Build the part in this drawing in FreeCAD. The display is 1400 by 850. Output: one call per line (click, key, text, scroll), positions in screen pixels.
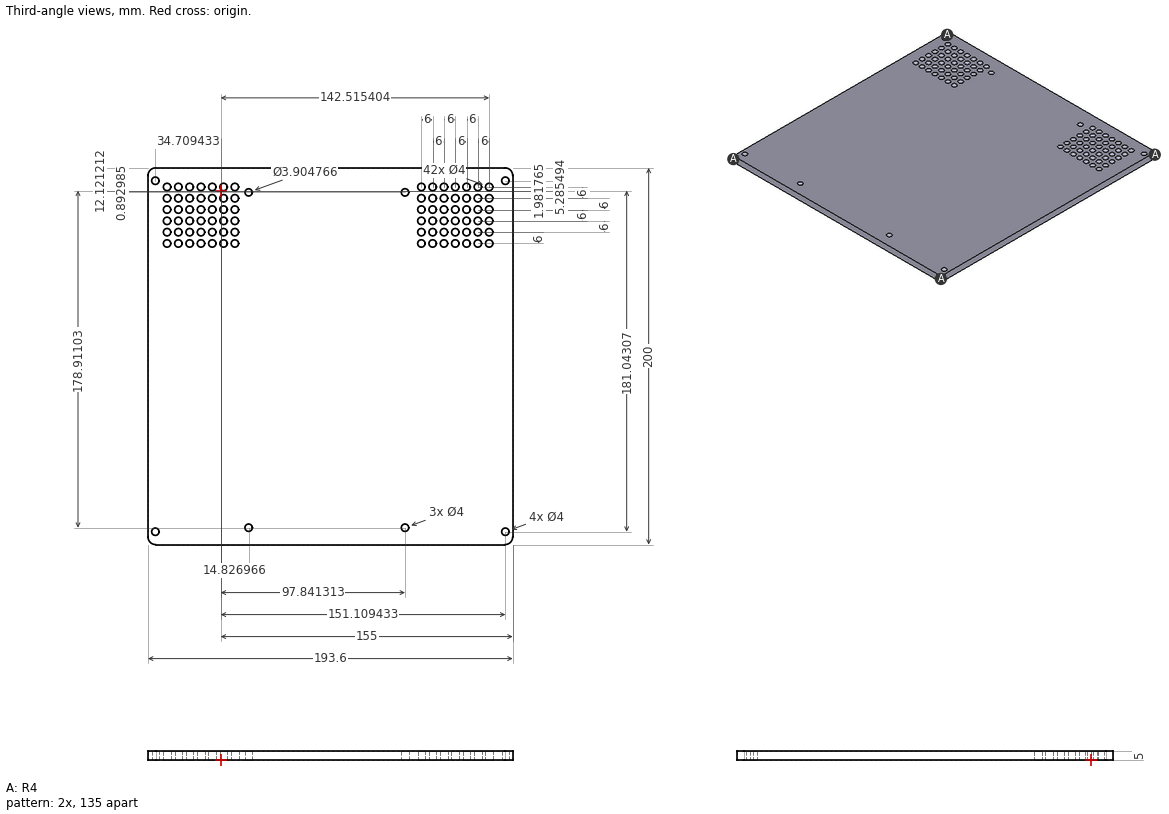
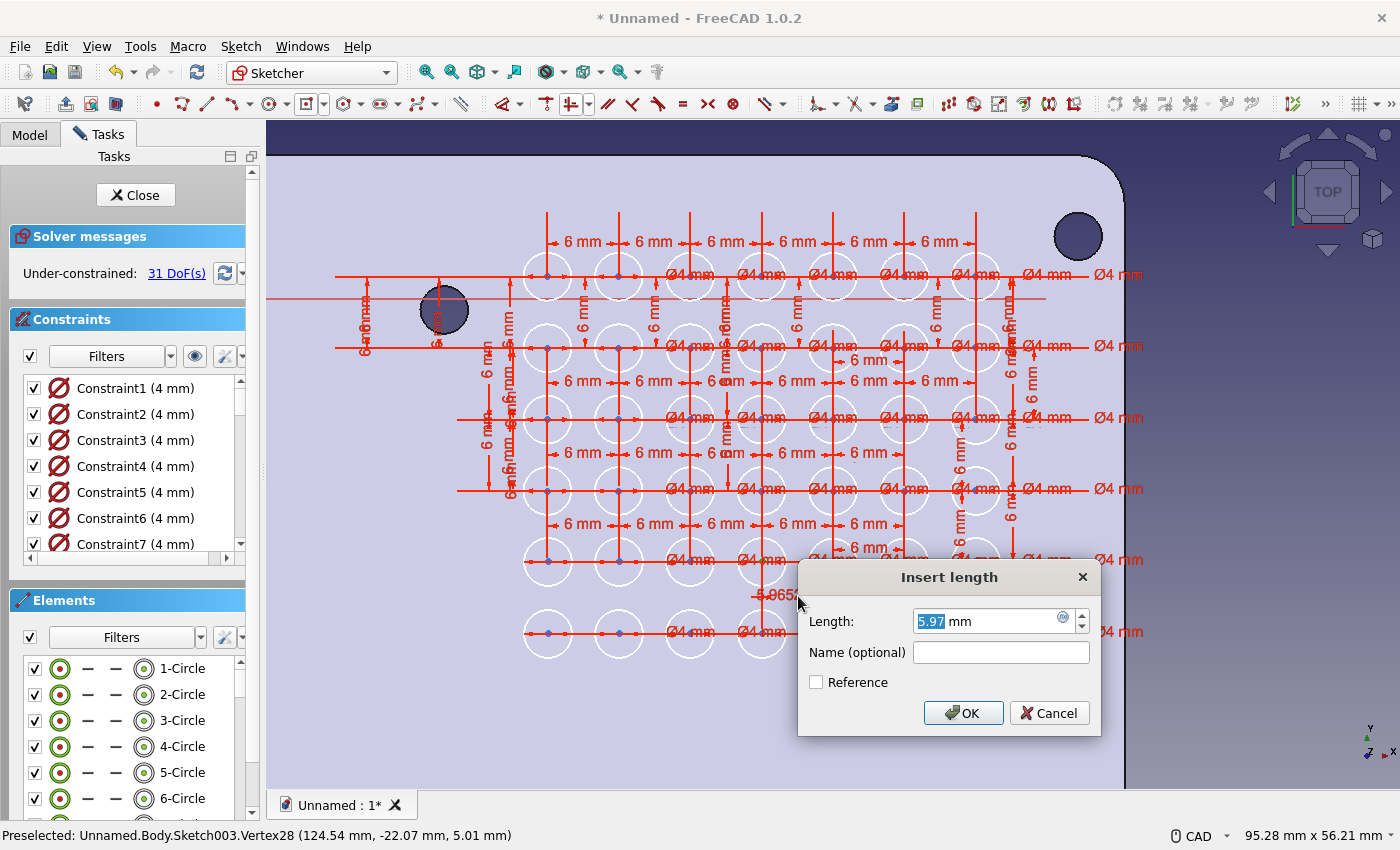
text(6)
key(Return)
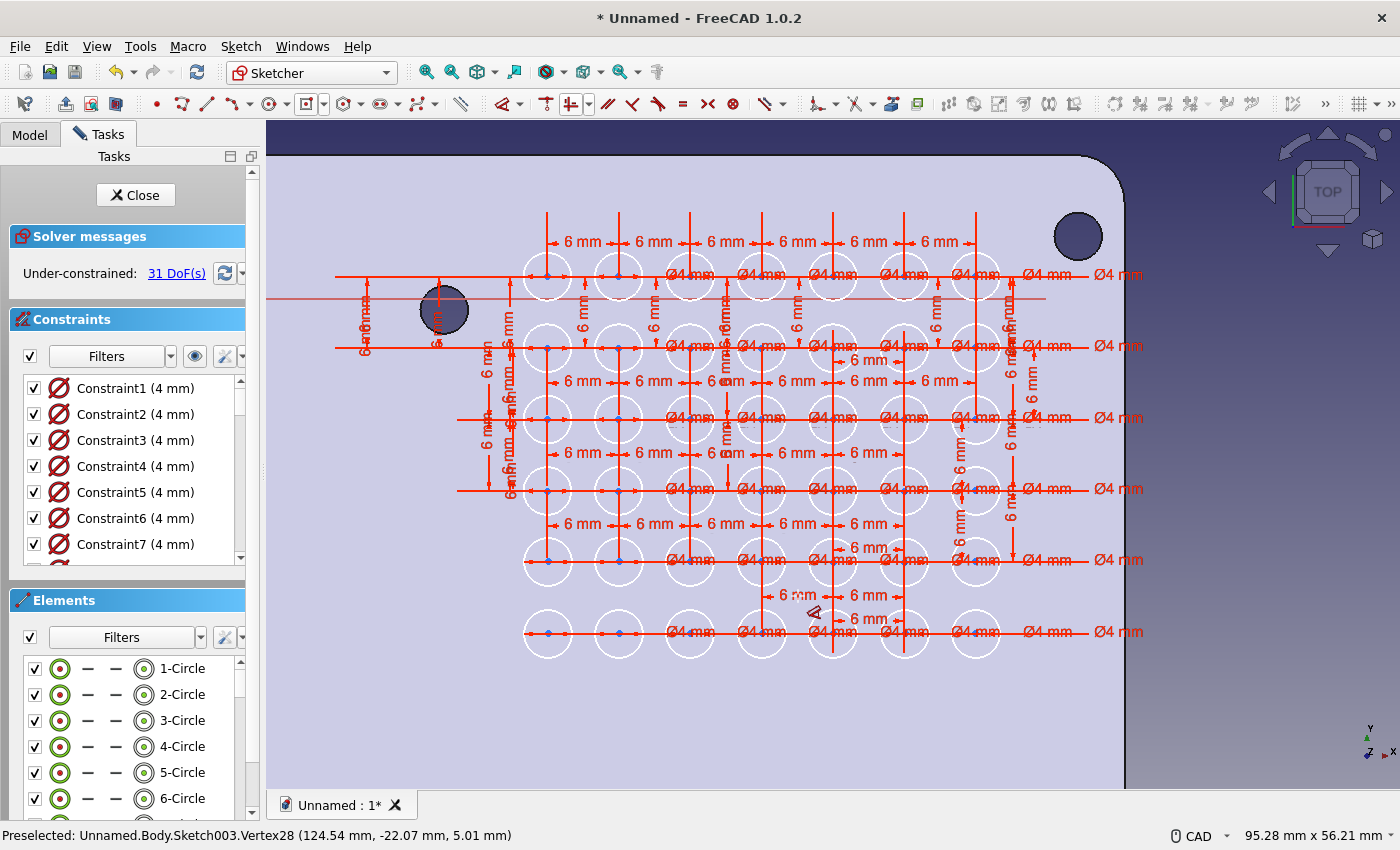
click(762, 491)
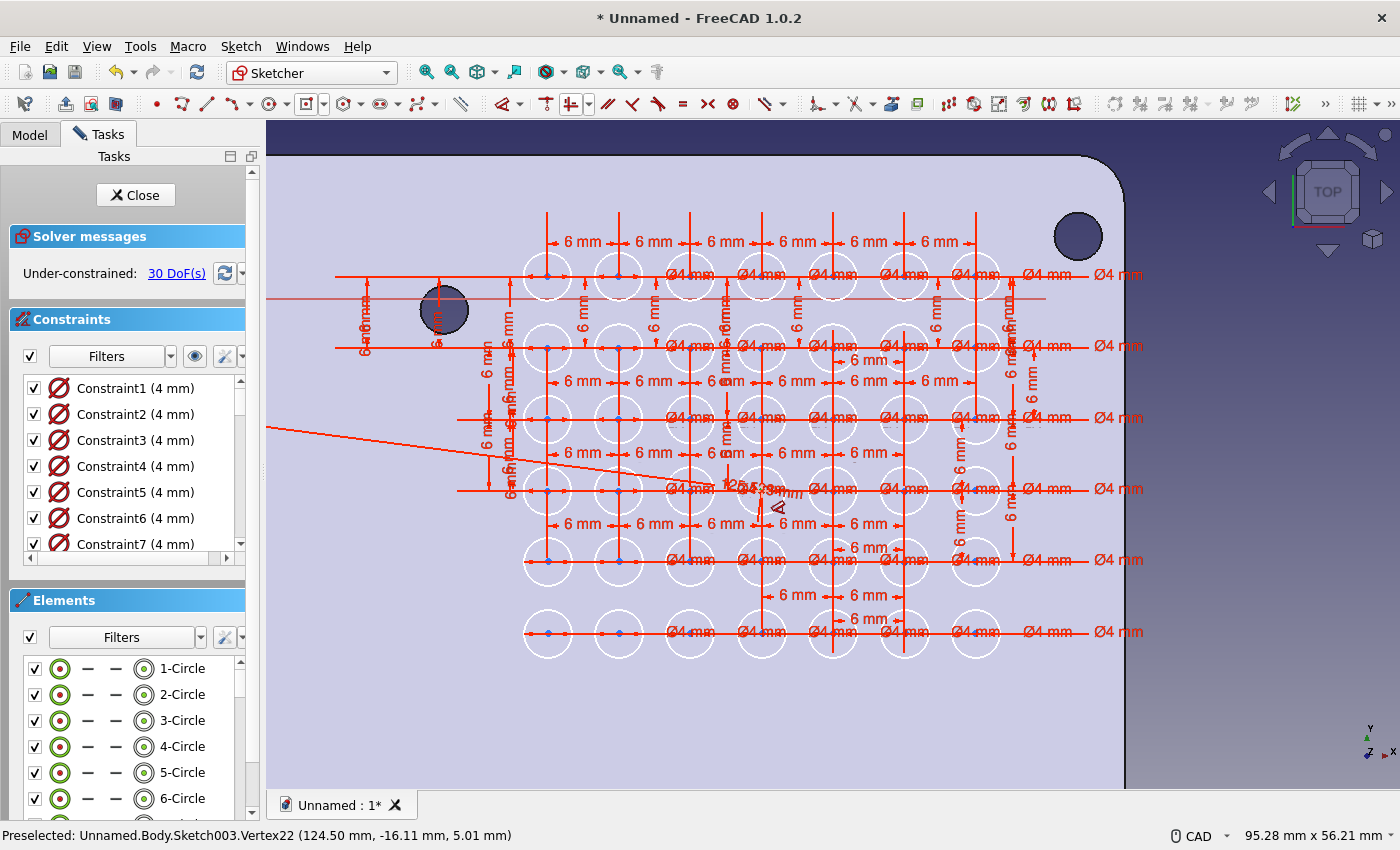
click(762, 562)
click(728, 510)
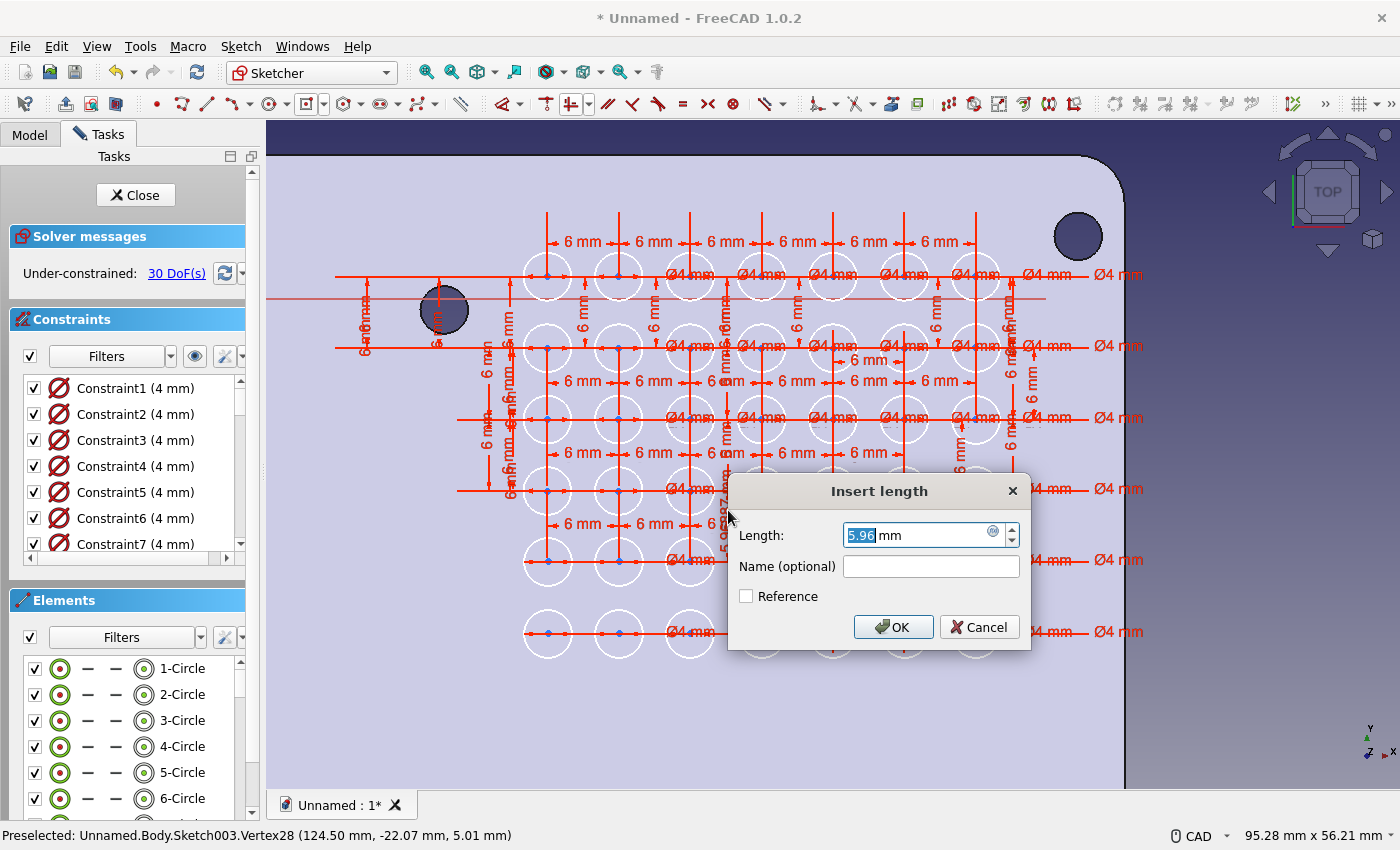
text(6)
key(Return)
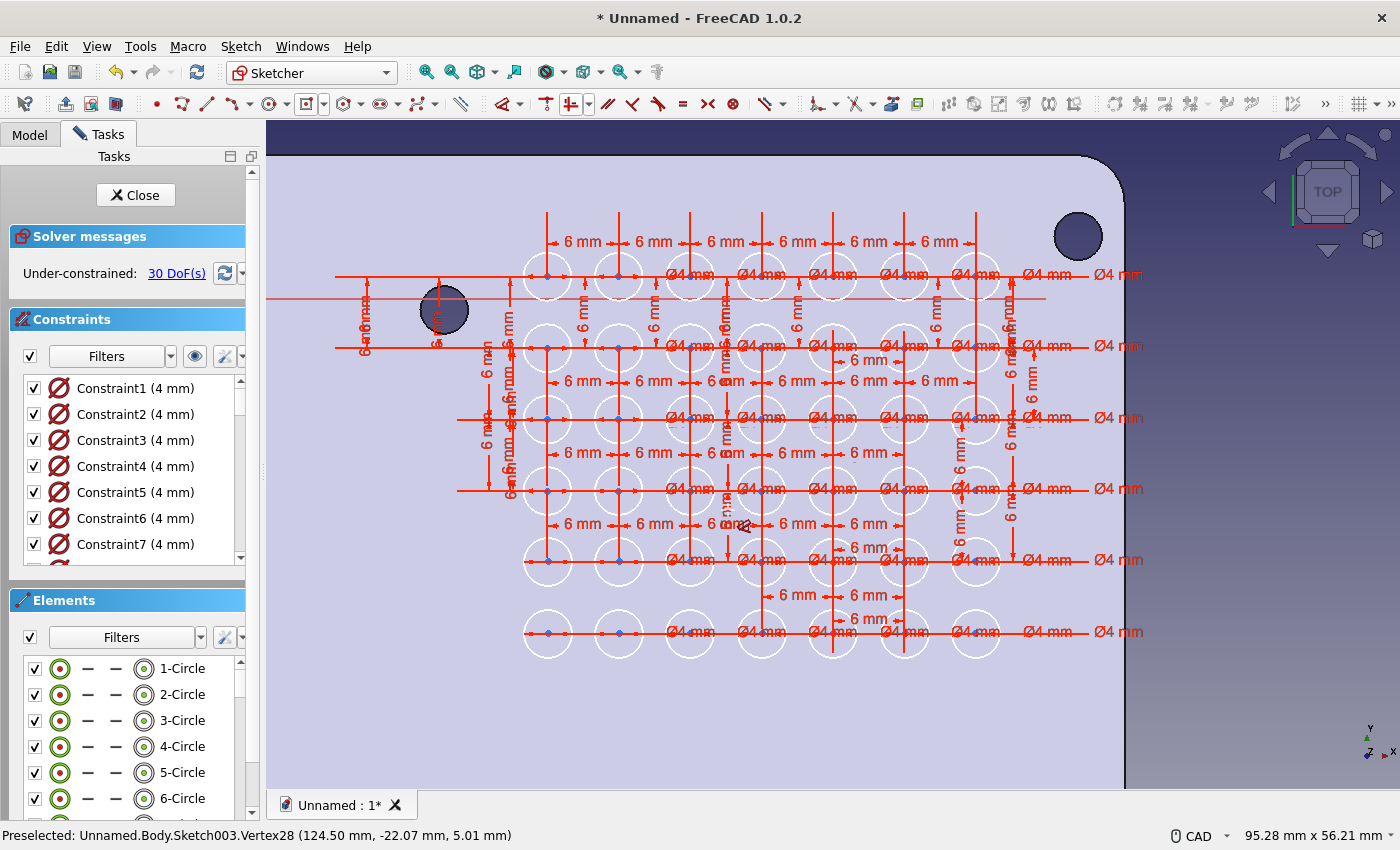
click(762, 562)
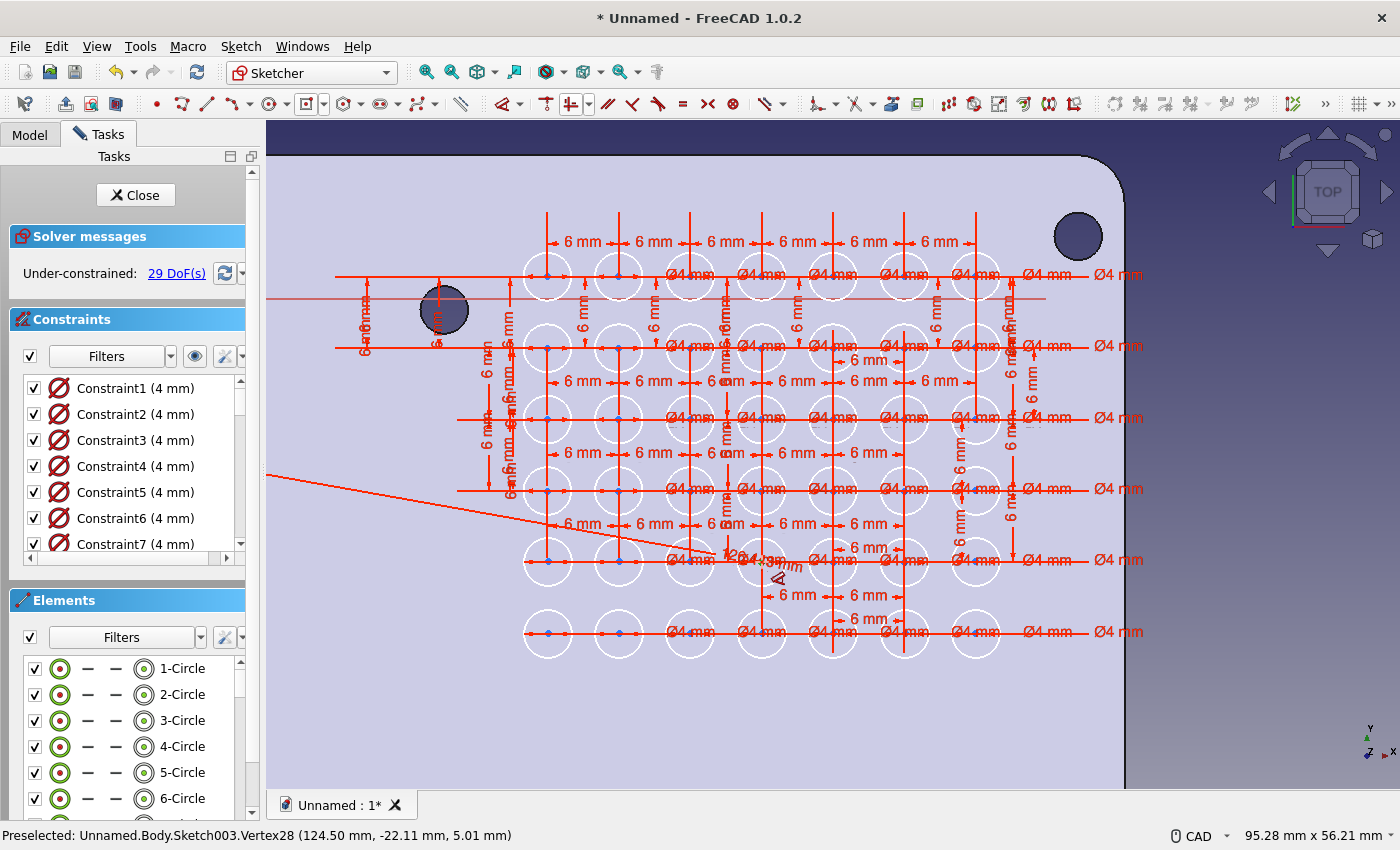
click(690, 562)
click(726, 596)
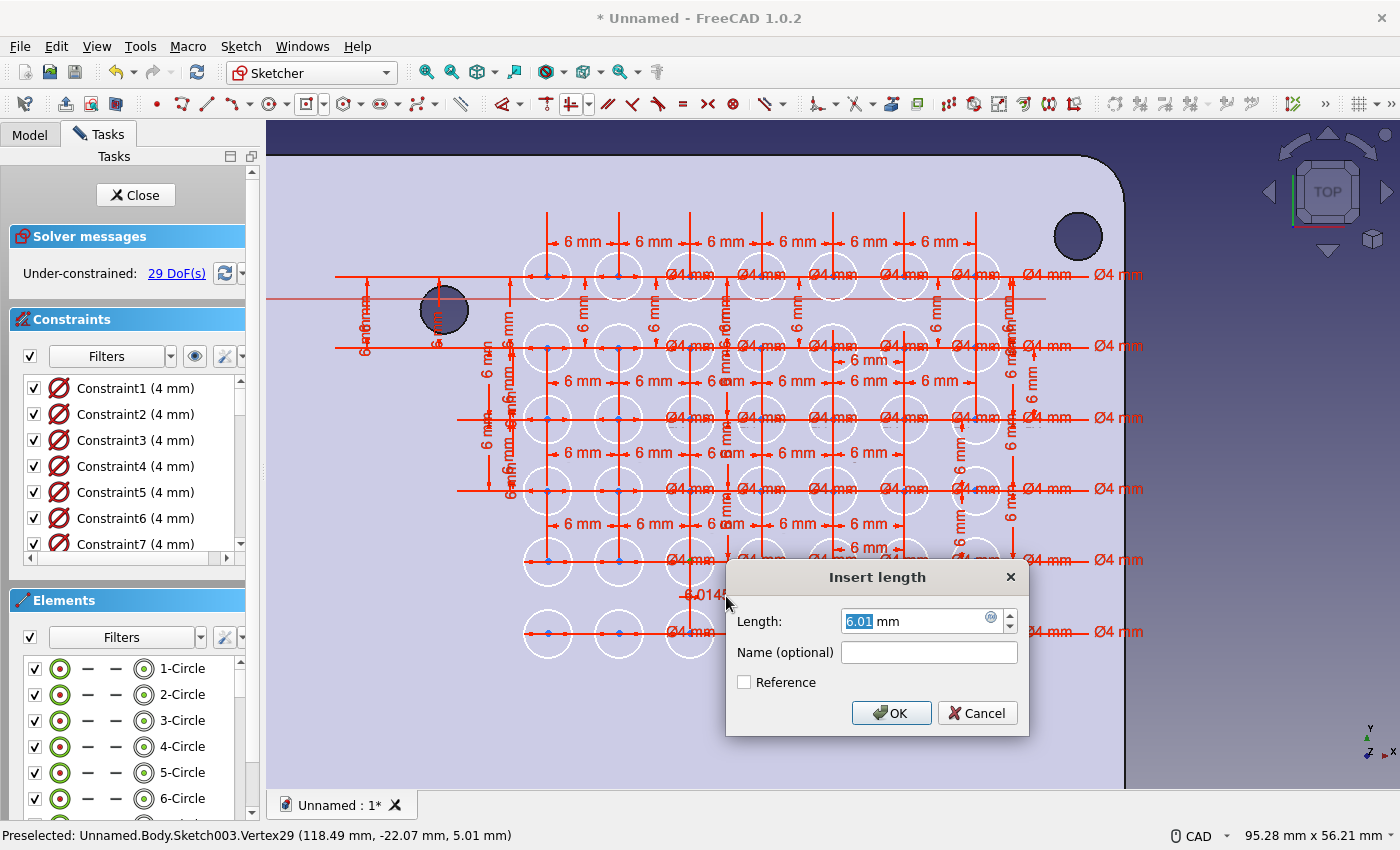
text(6)
key(Return)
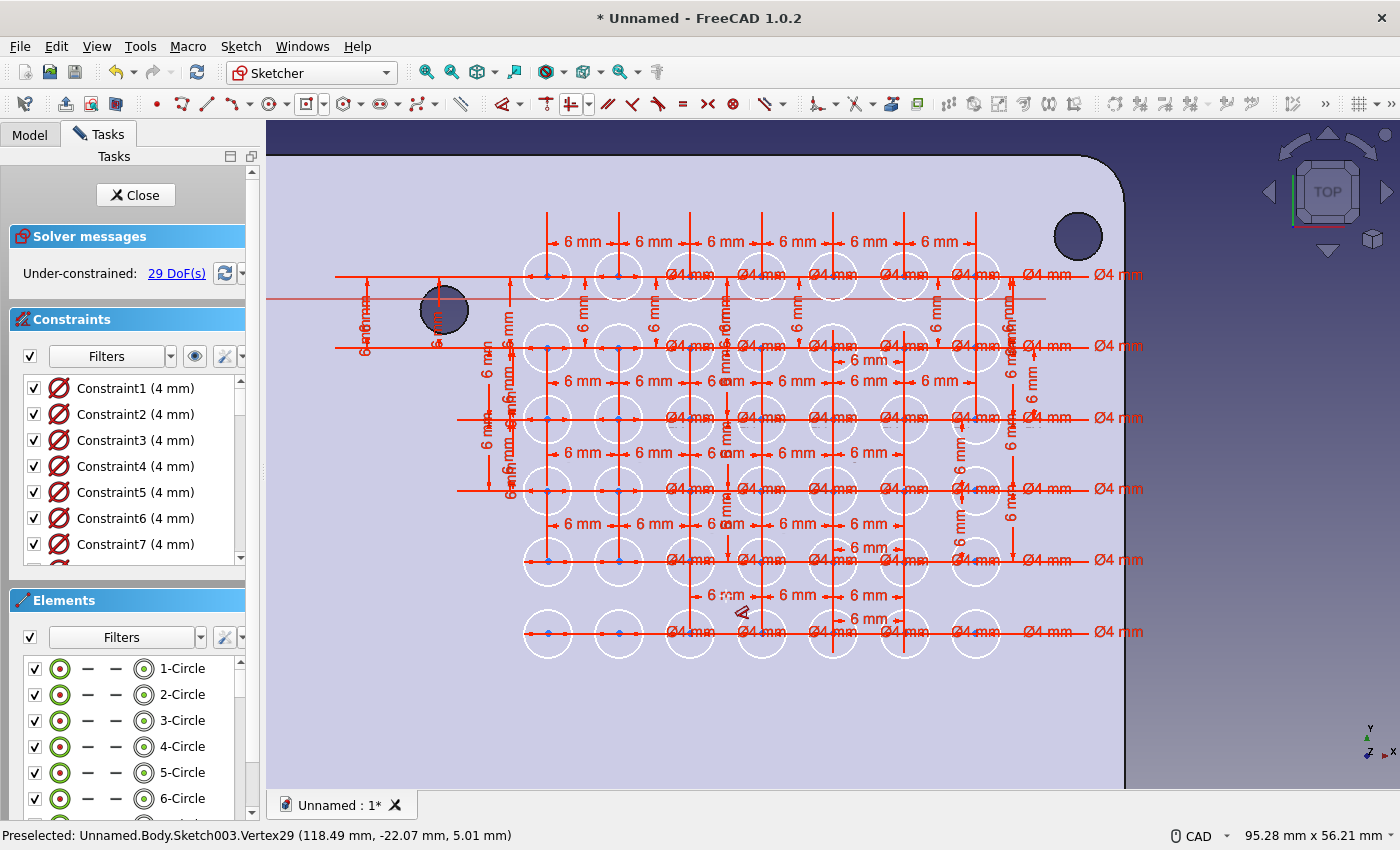
click(690, 491)